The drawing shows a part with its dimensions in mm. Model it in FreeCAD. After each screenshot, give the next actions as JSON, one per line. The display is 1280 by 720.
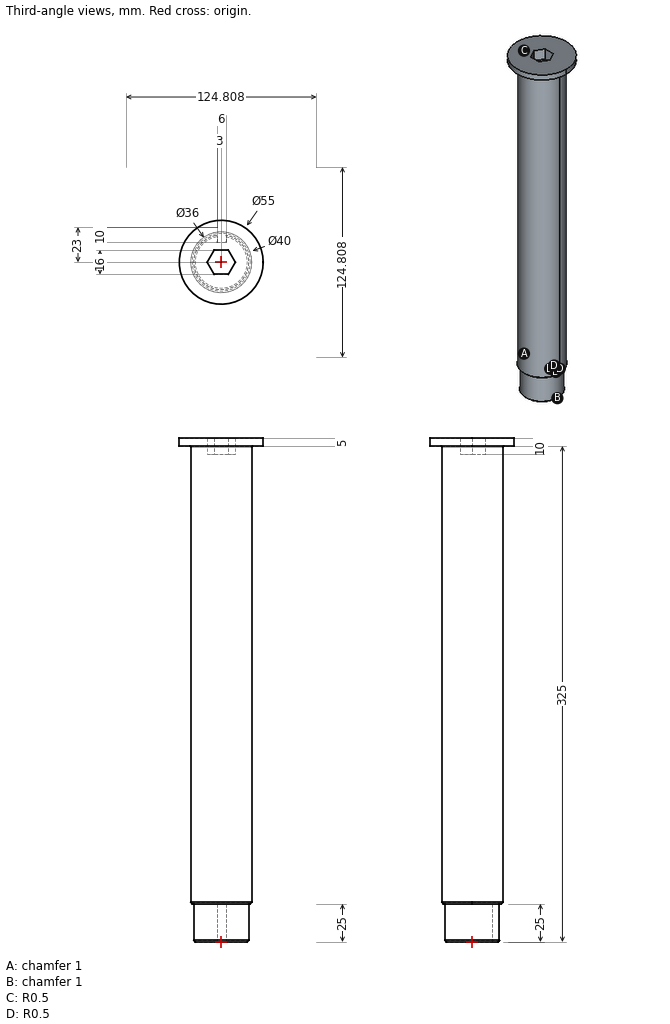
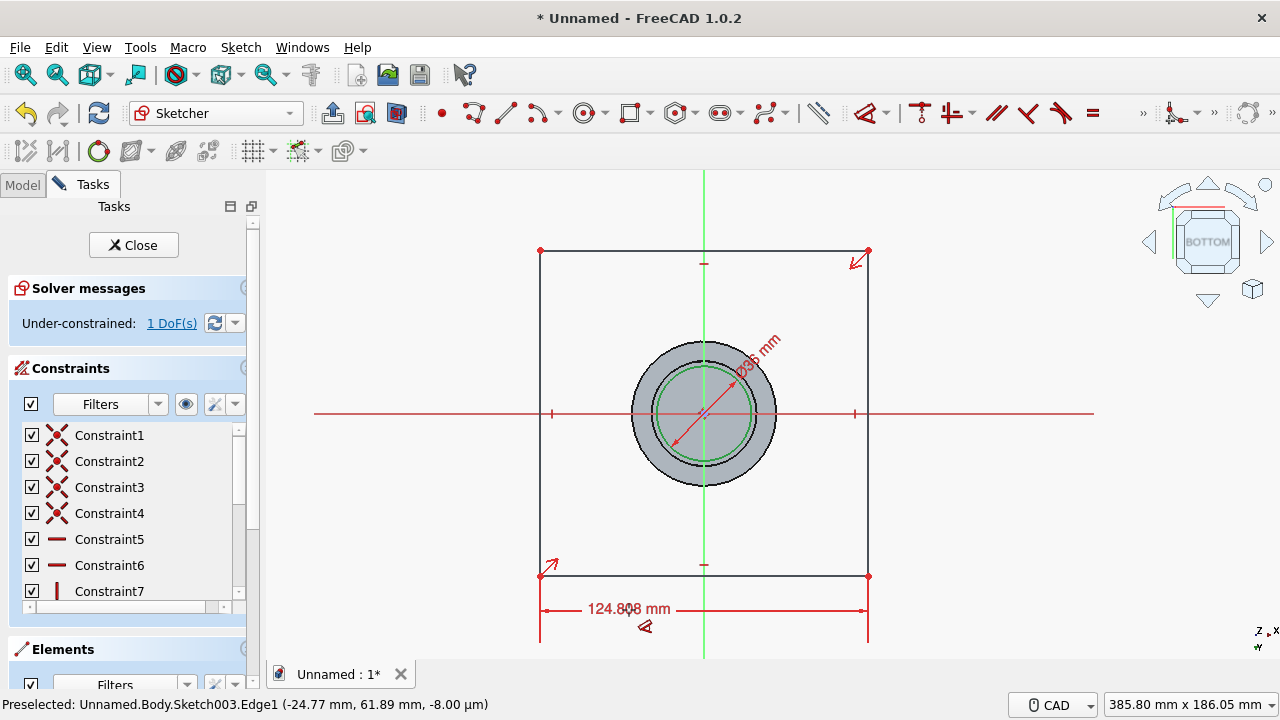
{"action": "left_click", "coordinate": [868, 479]}
{"action": "left_click", "coordinate": [902, 339]}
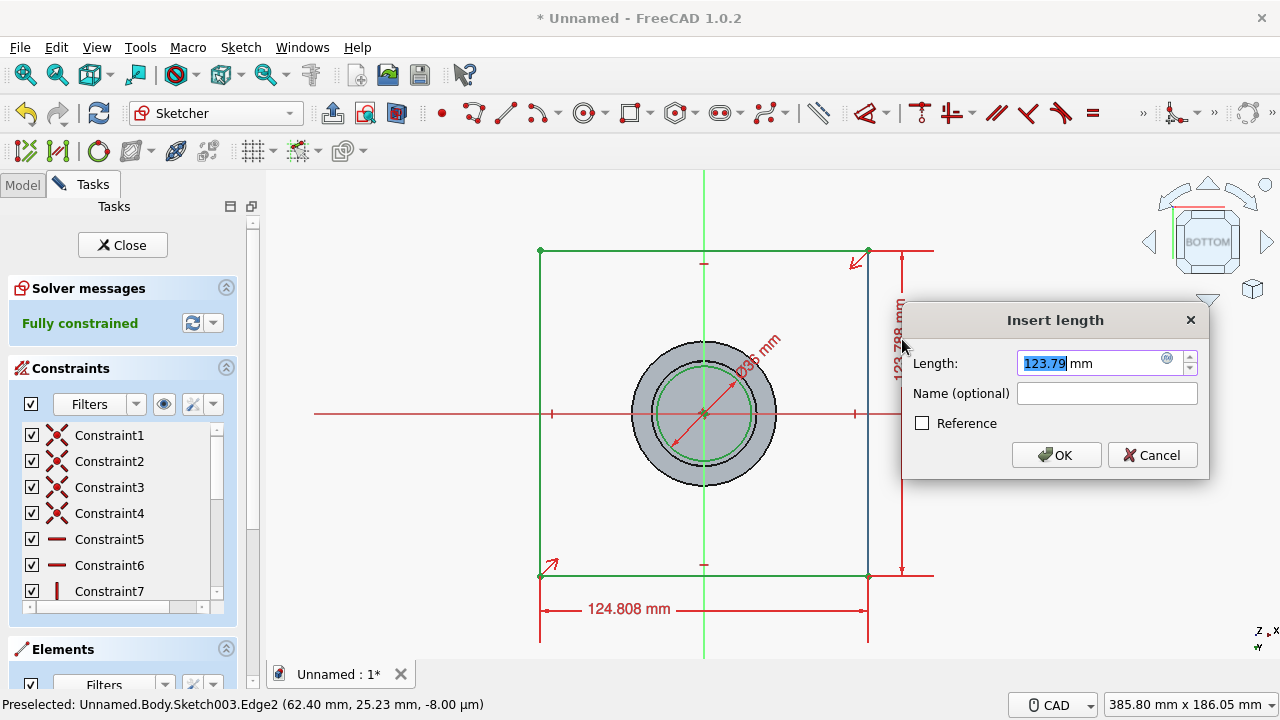
{"action": "type", "text": "124.808"}
{"action": "key", "text": "Return"}
{"action": "key", "text": "Escape"}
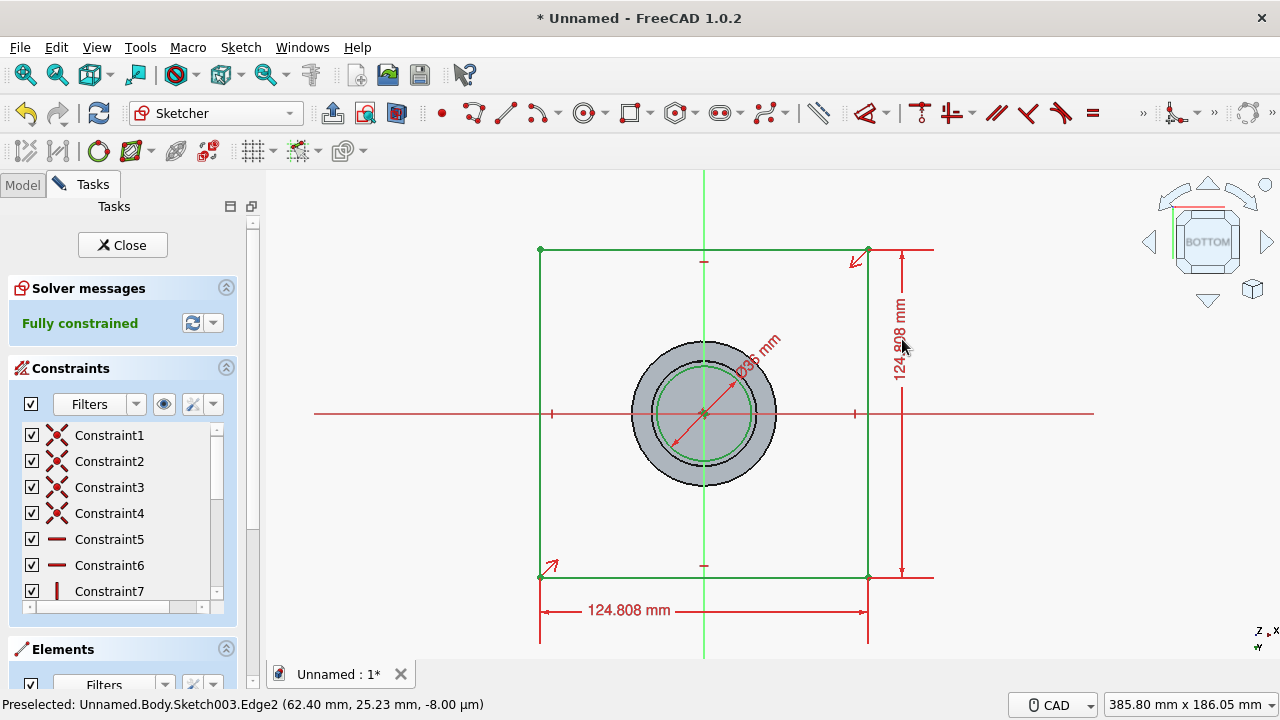
{"action": "left_click", "coordinate": [123, 245]}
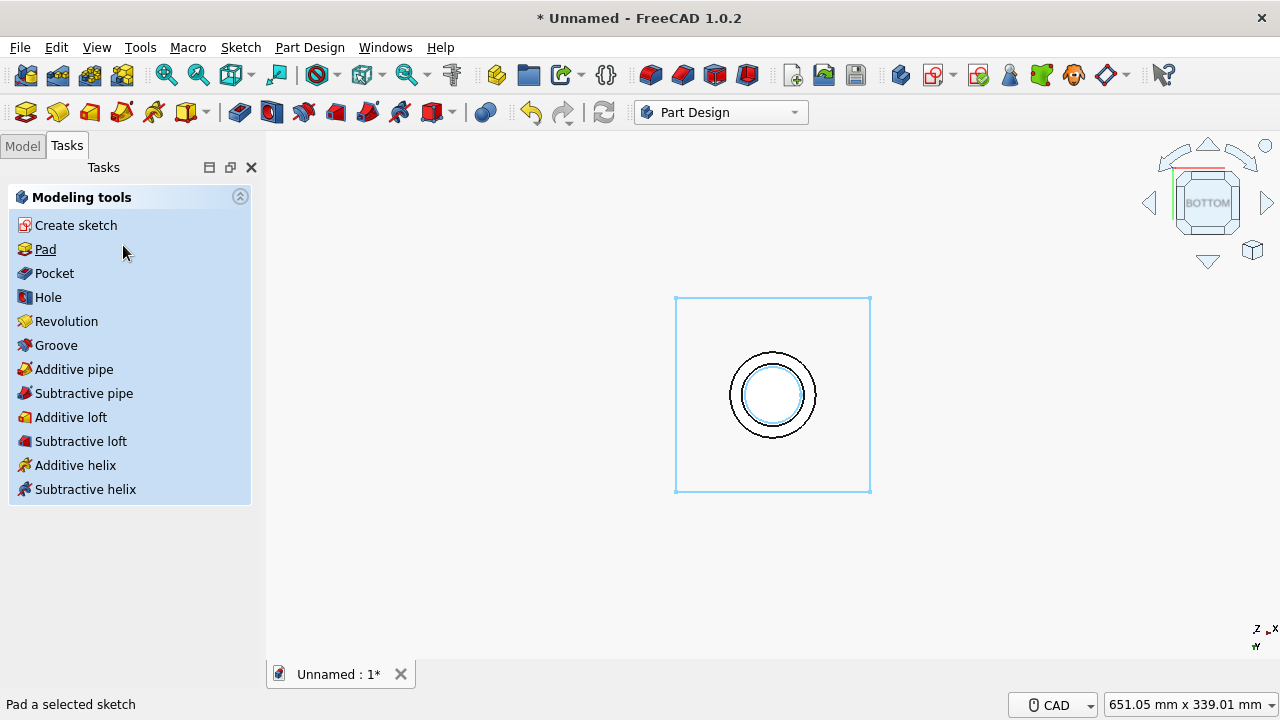
{"action": "left_click", "coordinate": [240, 112]}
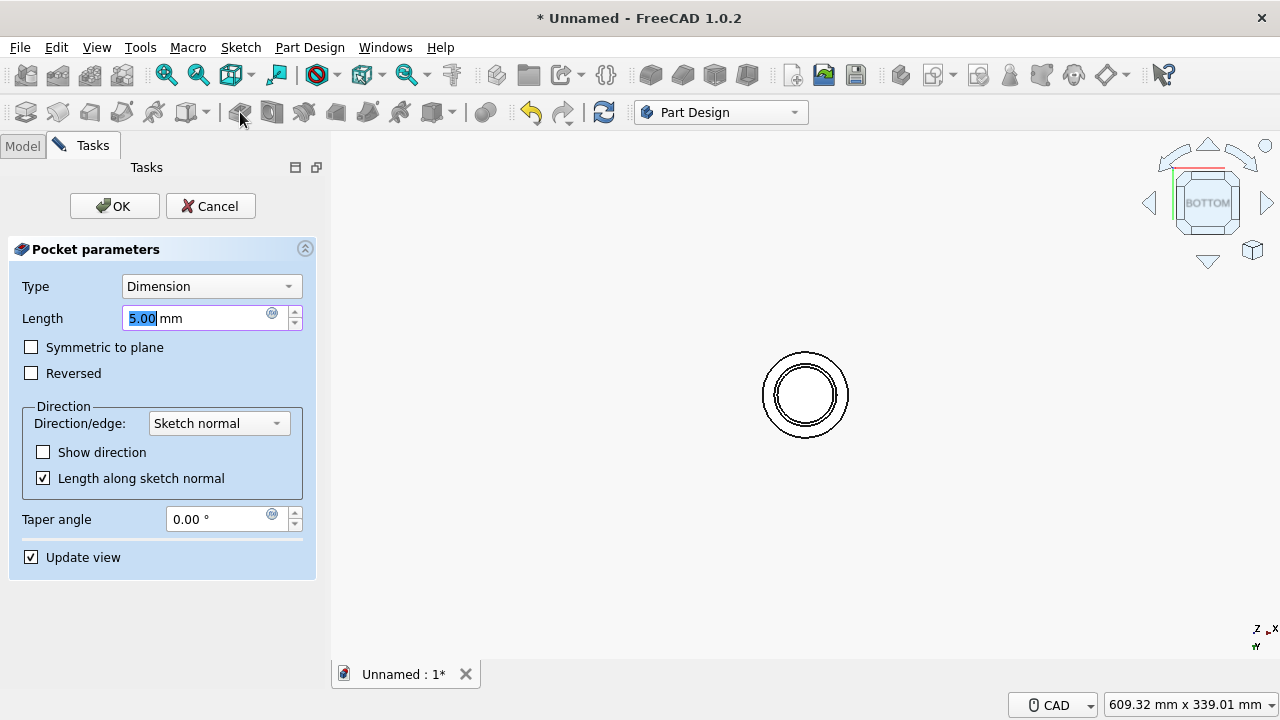
{"action": "type", "text": "25"}
{"action": "key", "text": "Tab"}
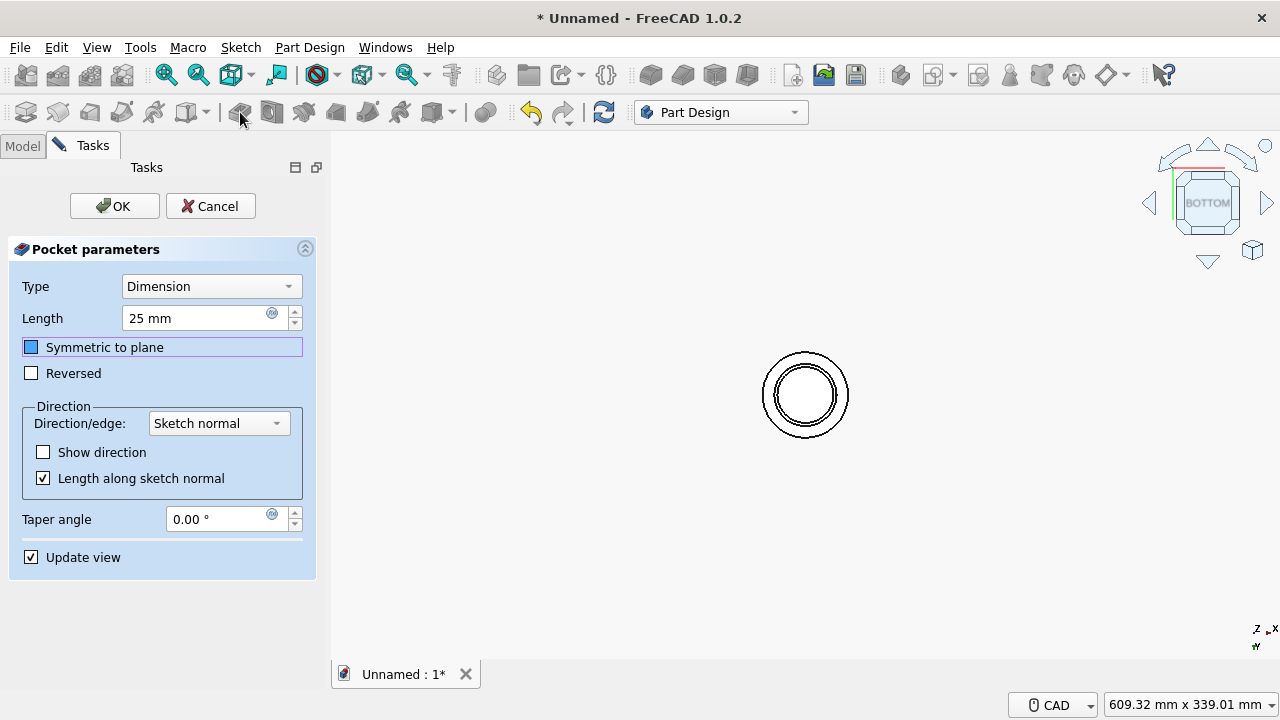
{"action": "left_click", "coordinate": [115, 206]}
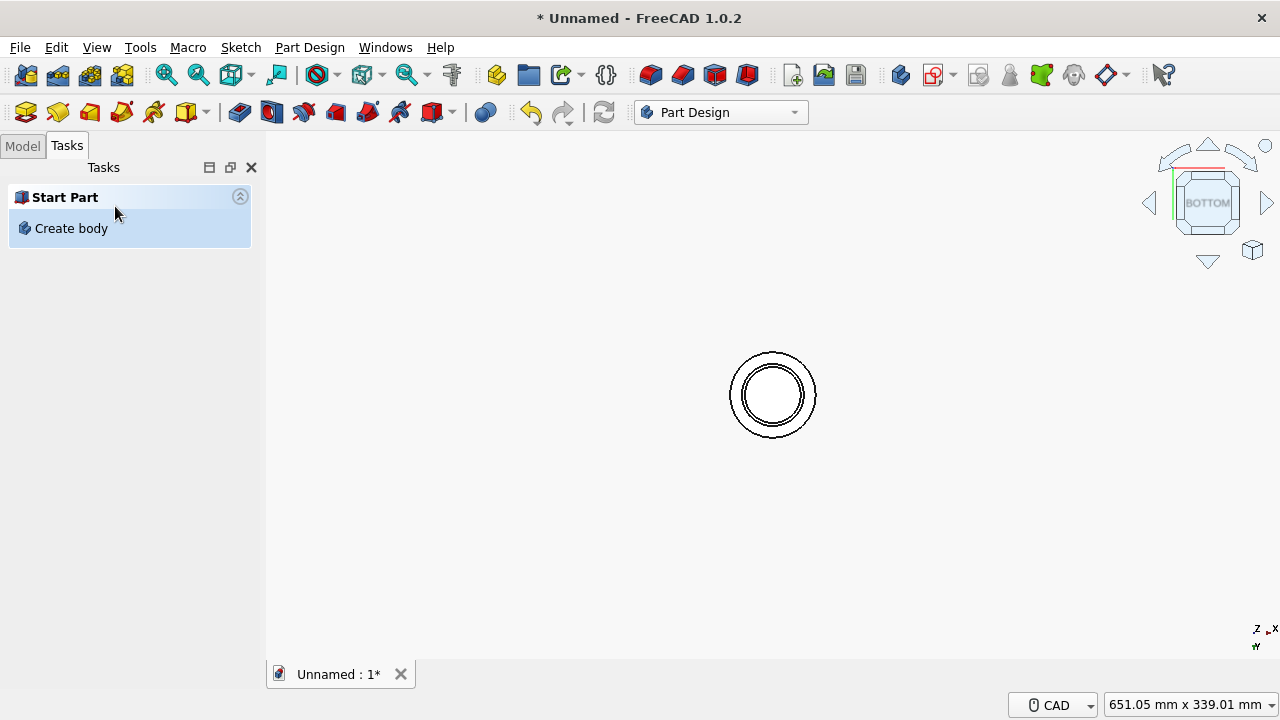
{"action": "left_click", "coordinate": [168, 76]}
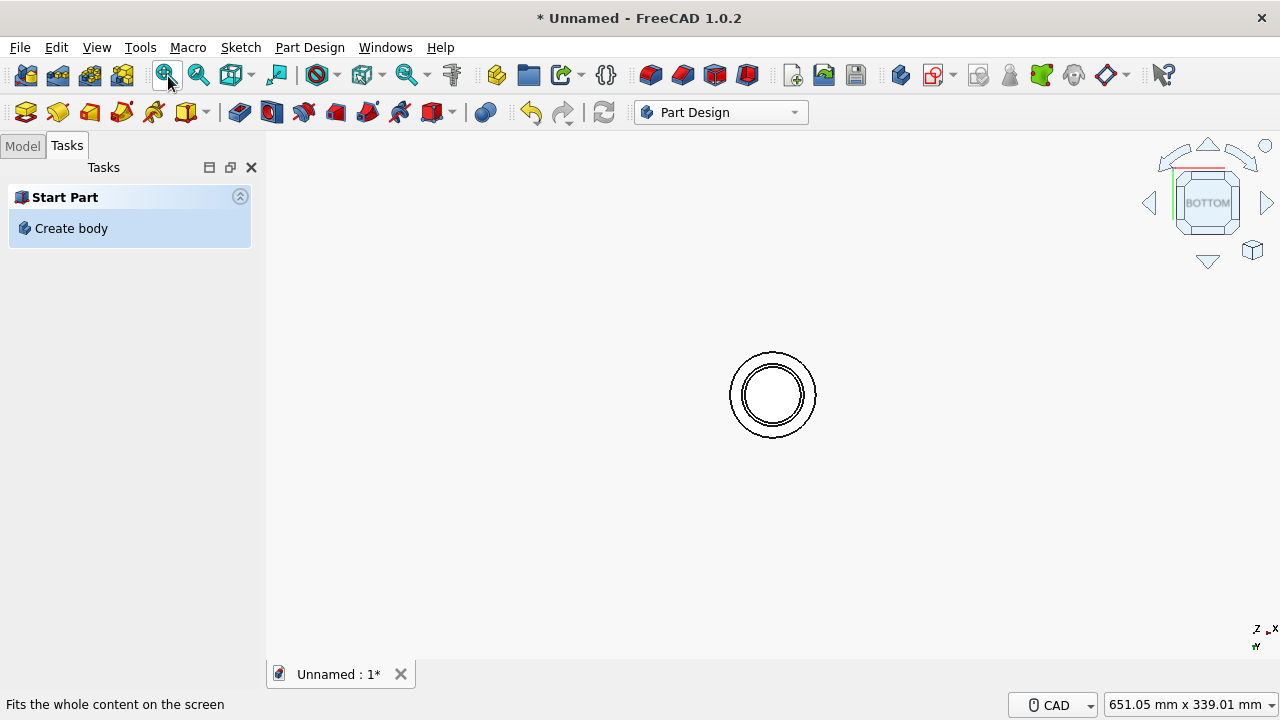
{"action": "key", "text": "0"}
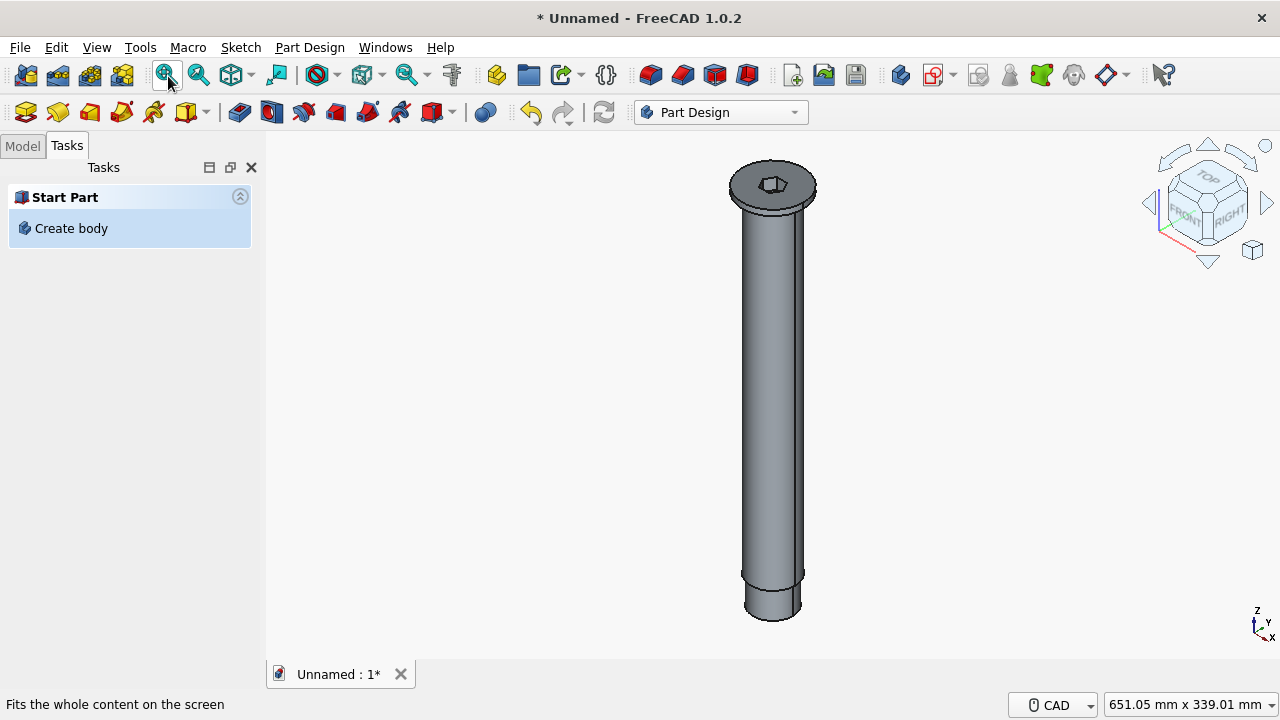
{"action": "key", "text": "2"}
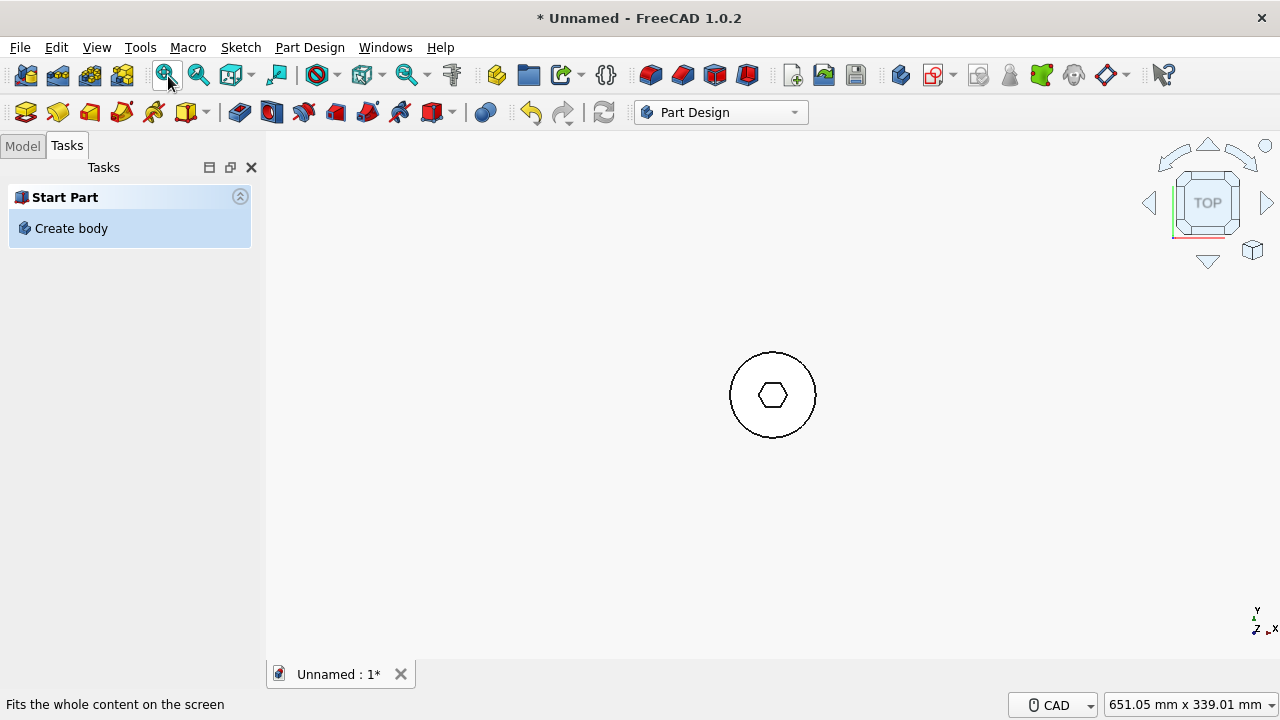
{"action": "left_click", "coordinate": [168, 76]}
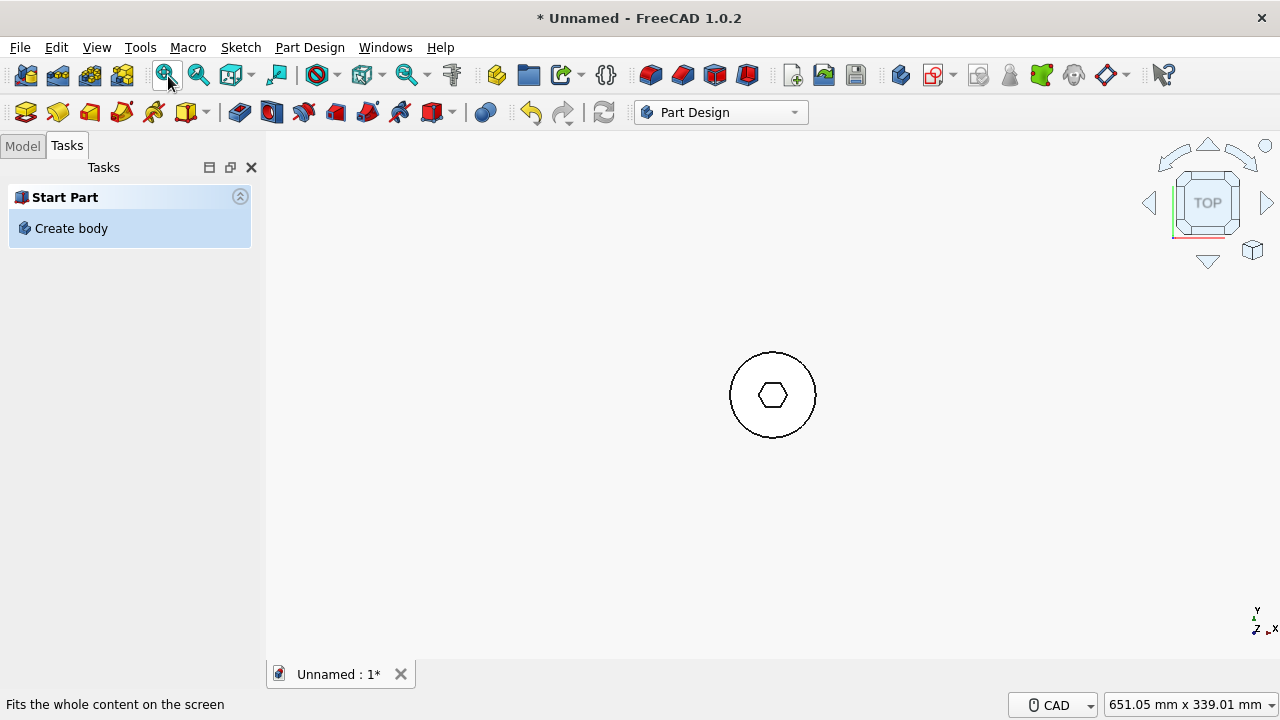
{"action": "key", "text": "1"}